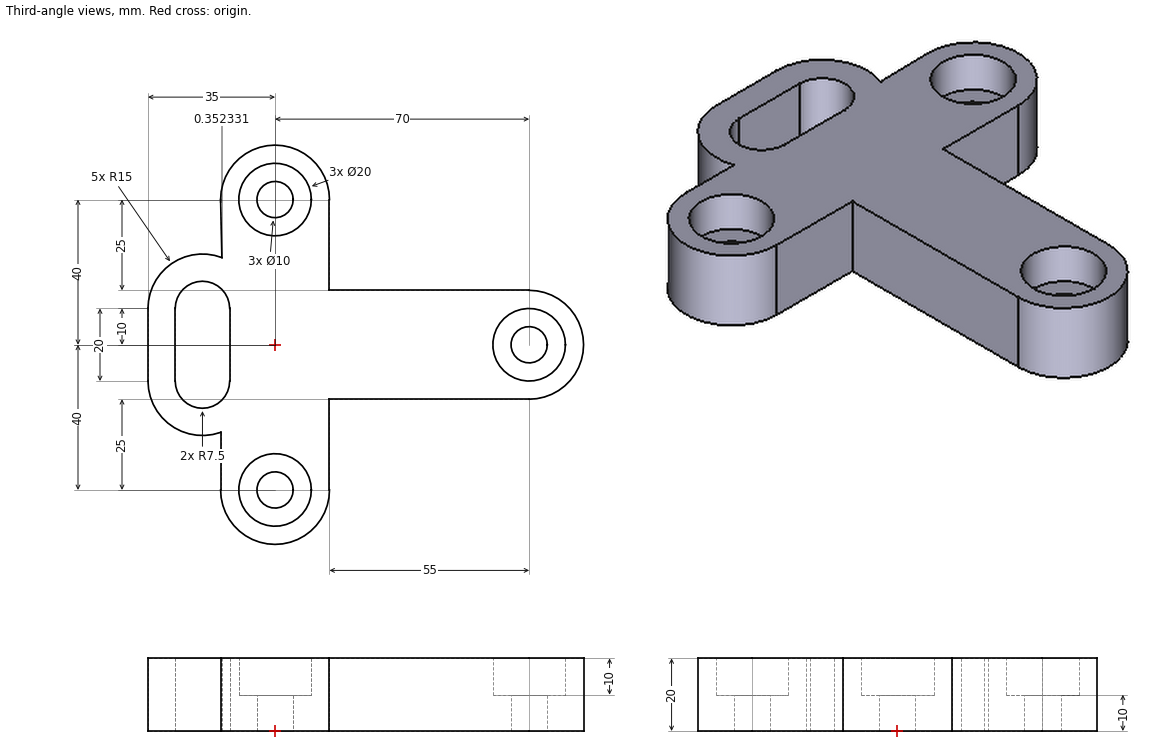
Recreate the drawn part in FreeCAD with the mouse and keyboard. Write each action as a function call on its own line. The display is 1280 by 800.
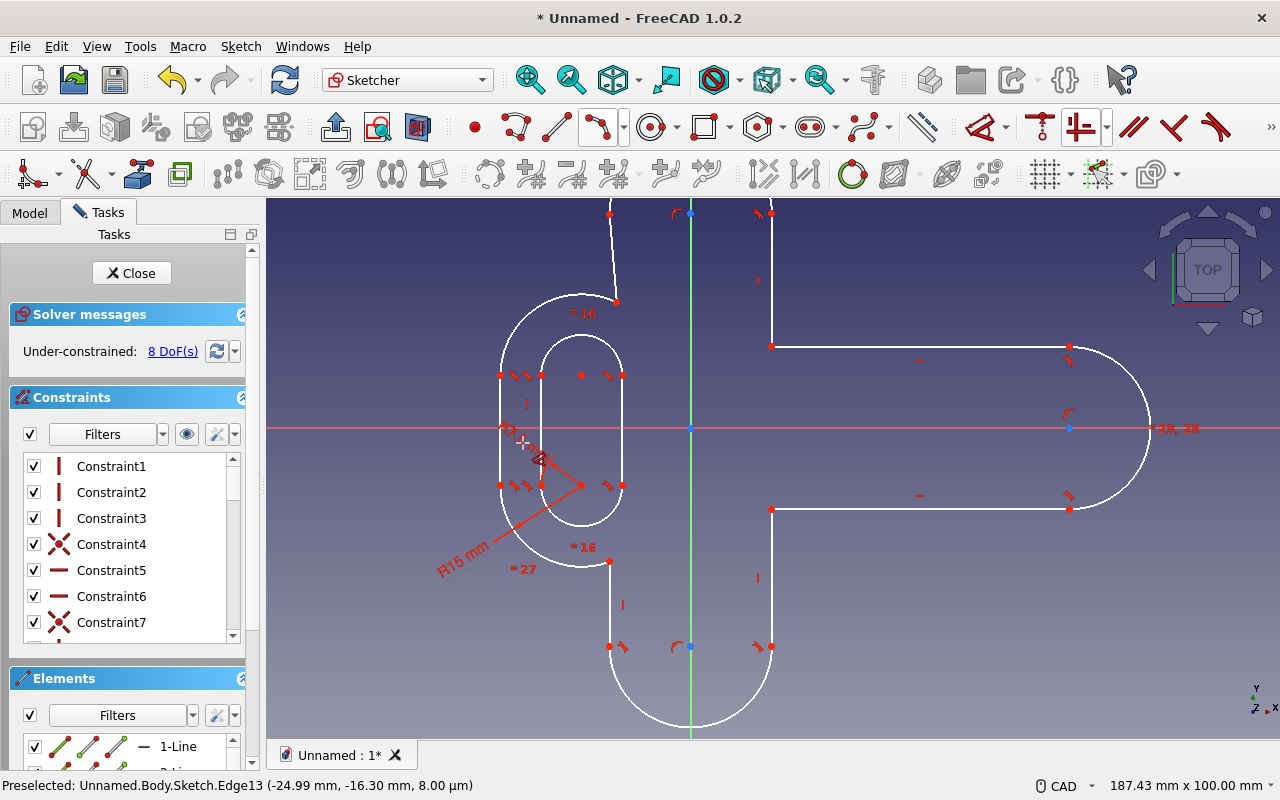
click(500, 409)
click(466, 405)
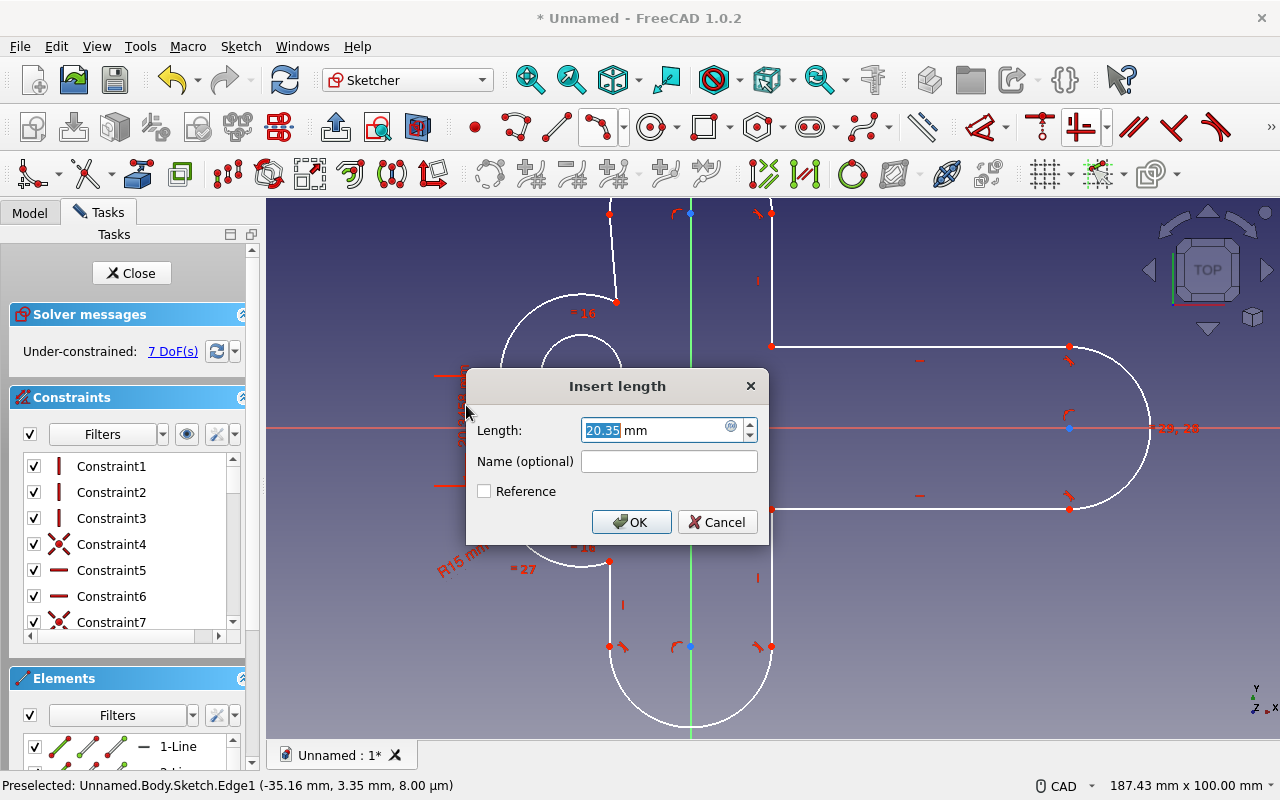
text(20)
key(Return)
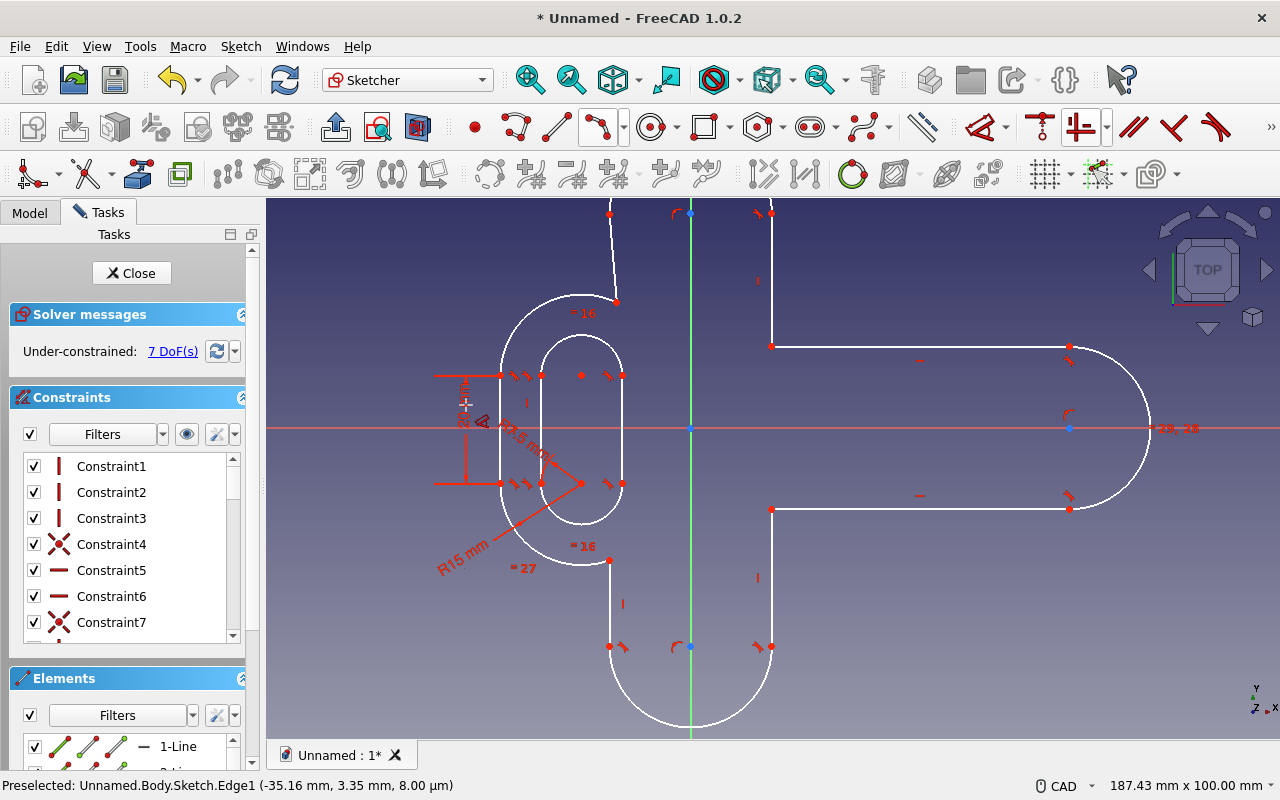
click(772, 605)
click(738, 578)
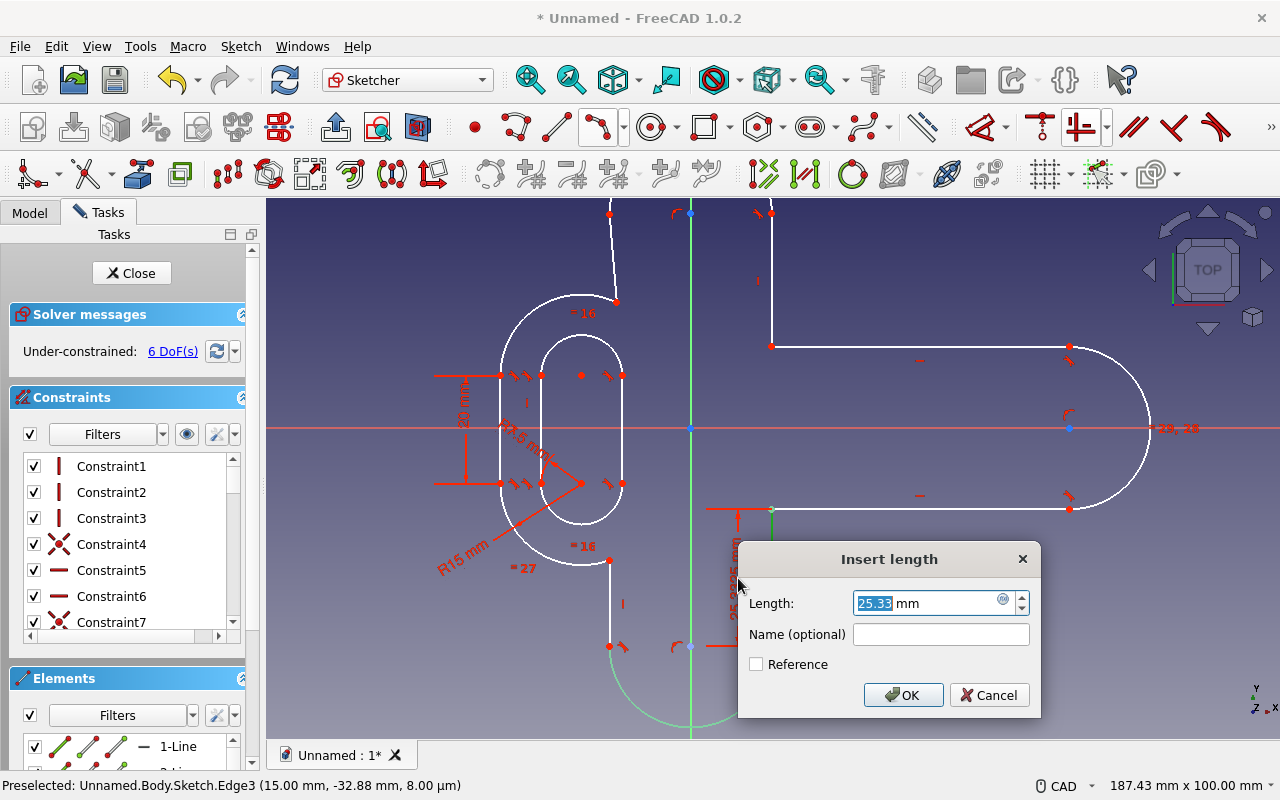
text(25)
key(Return)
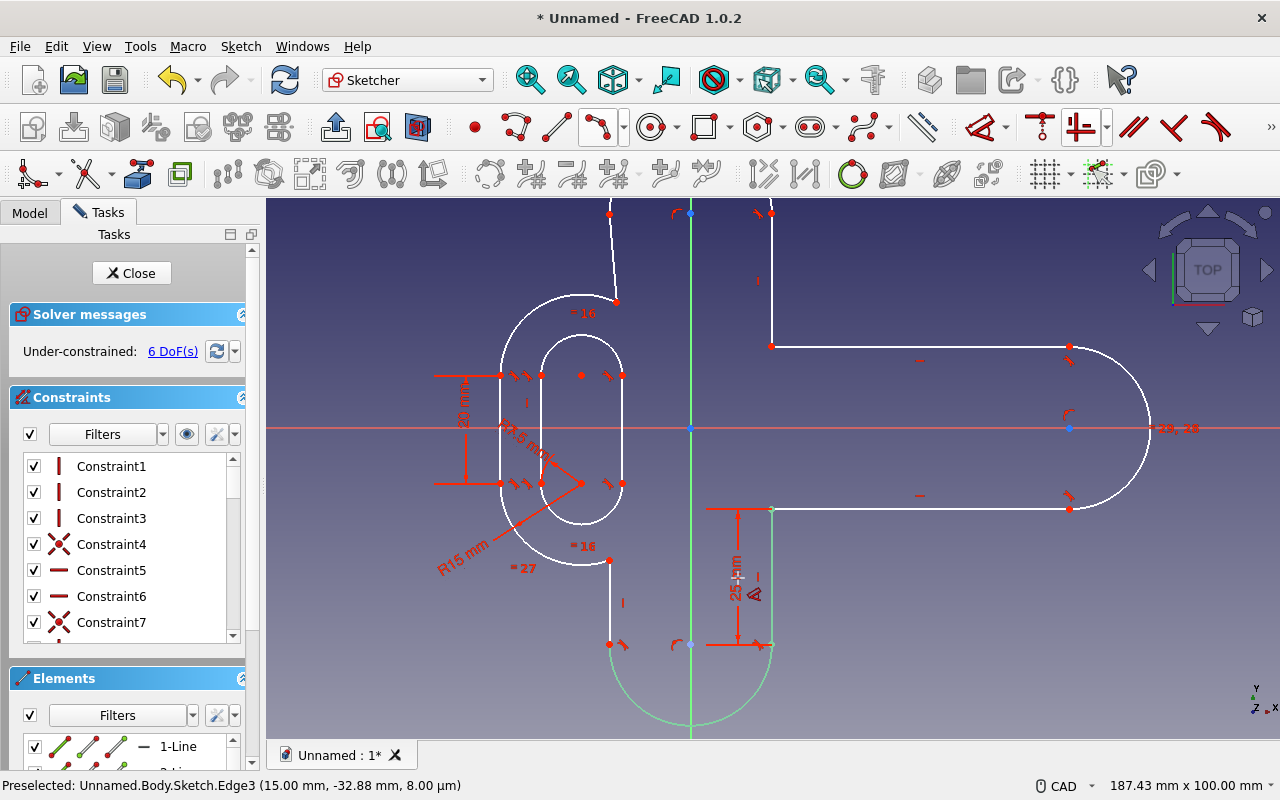
click(861, 509)
click(921, 543)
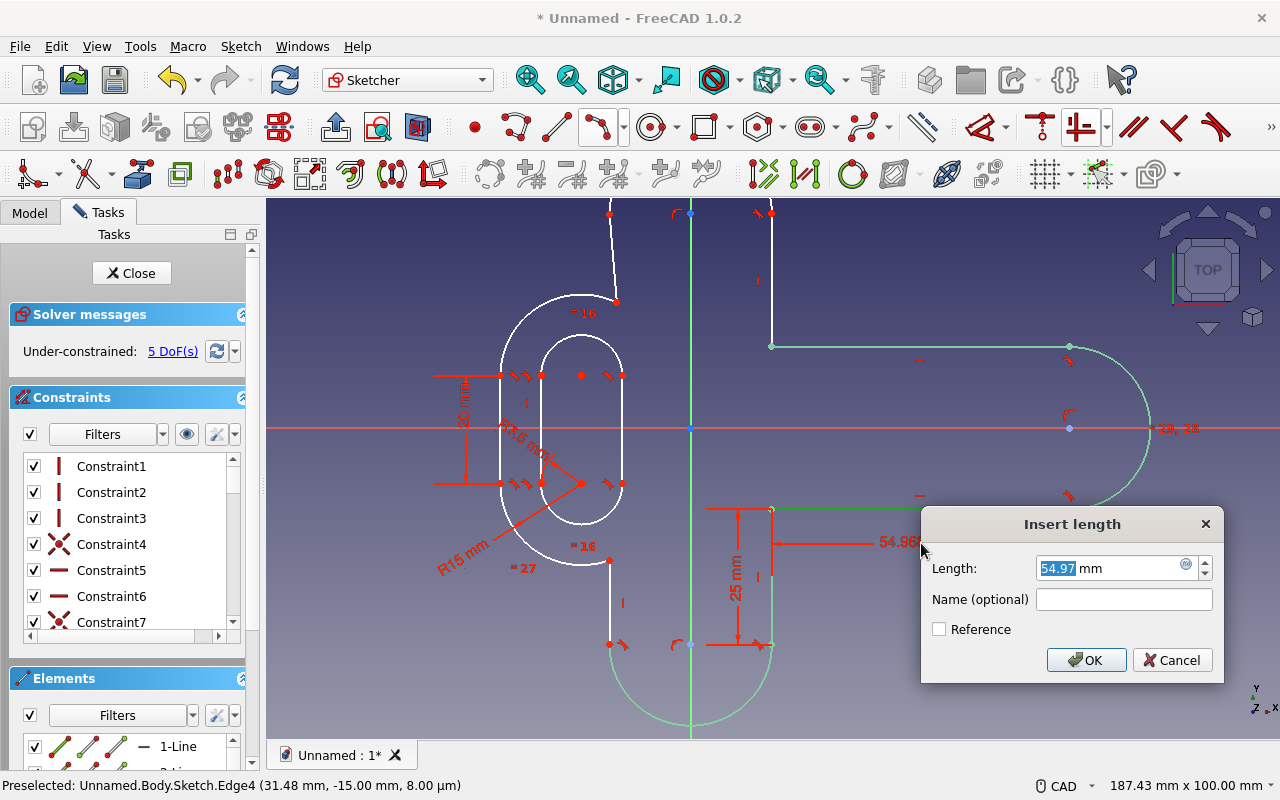
text(55)
key(Return)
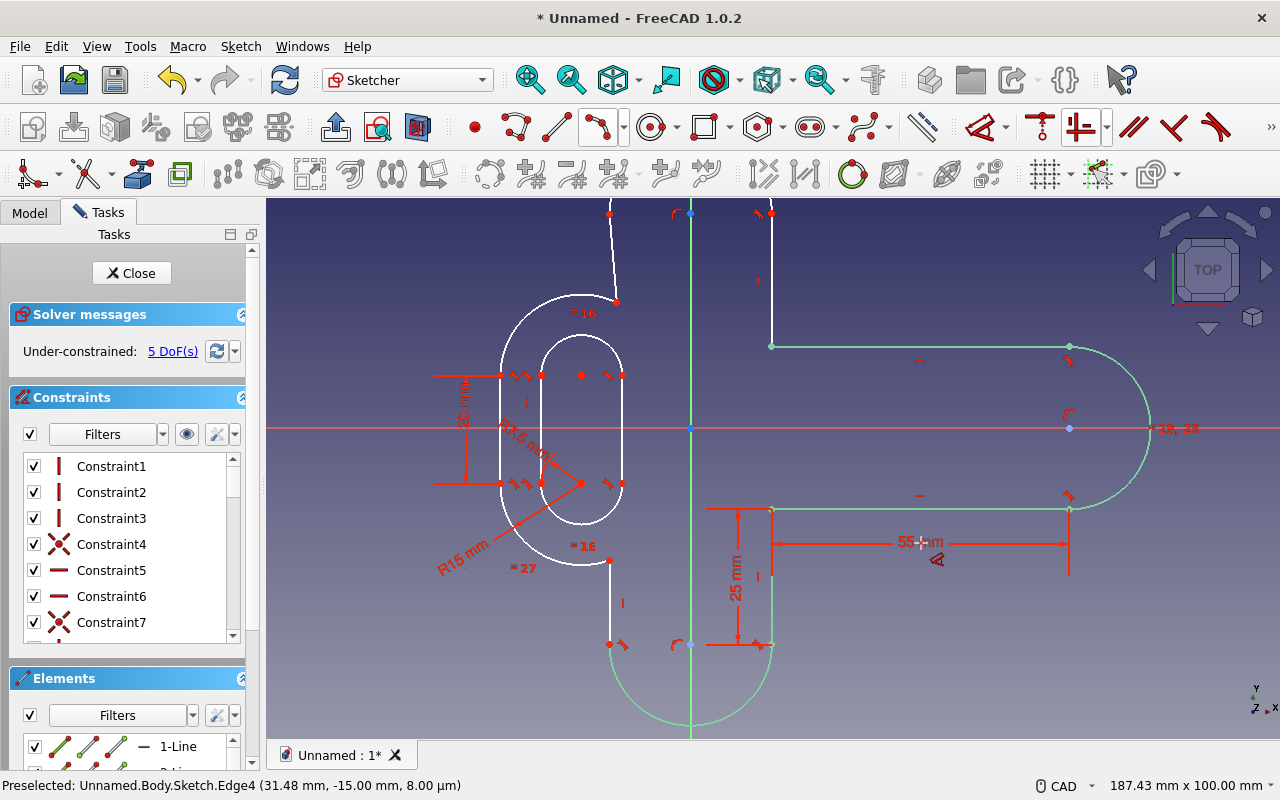
click(772, 307)
click(738, 286)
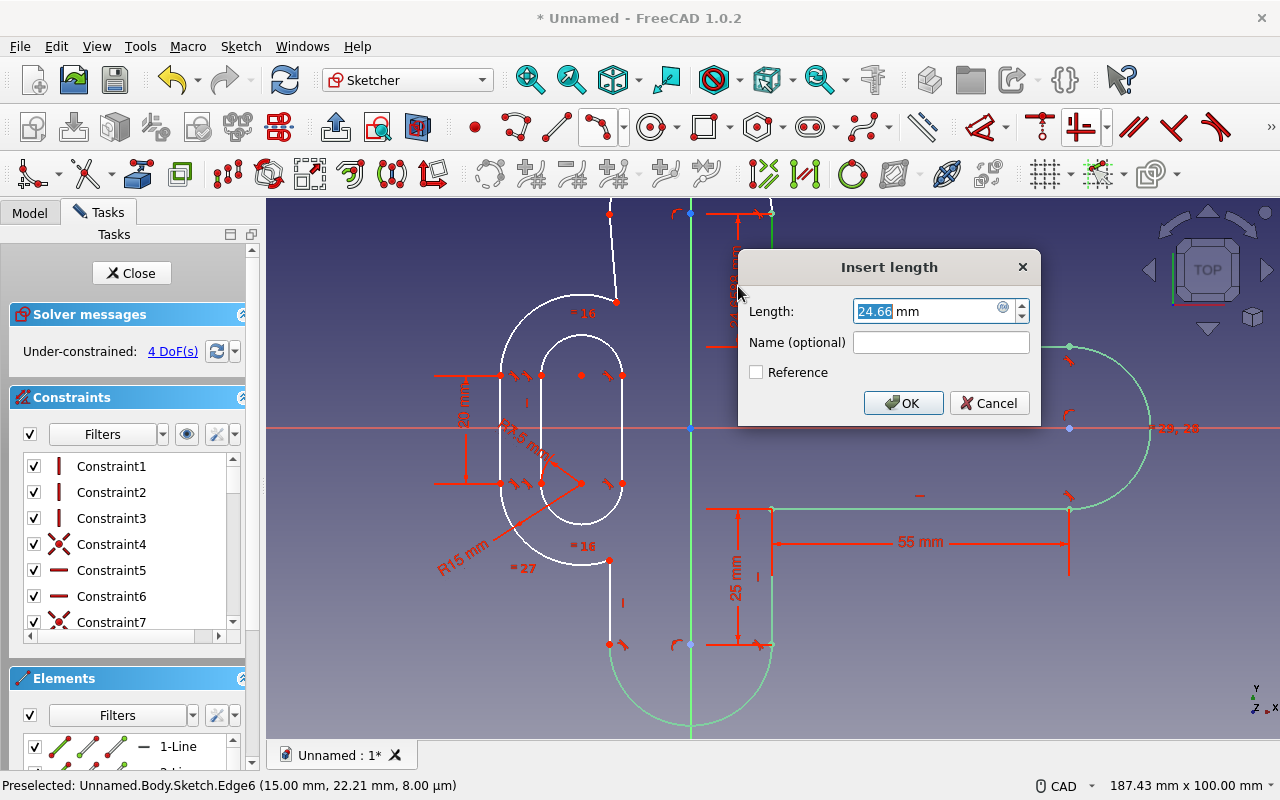
text(25)
key(Return)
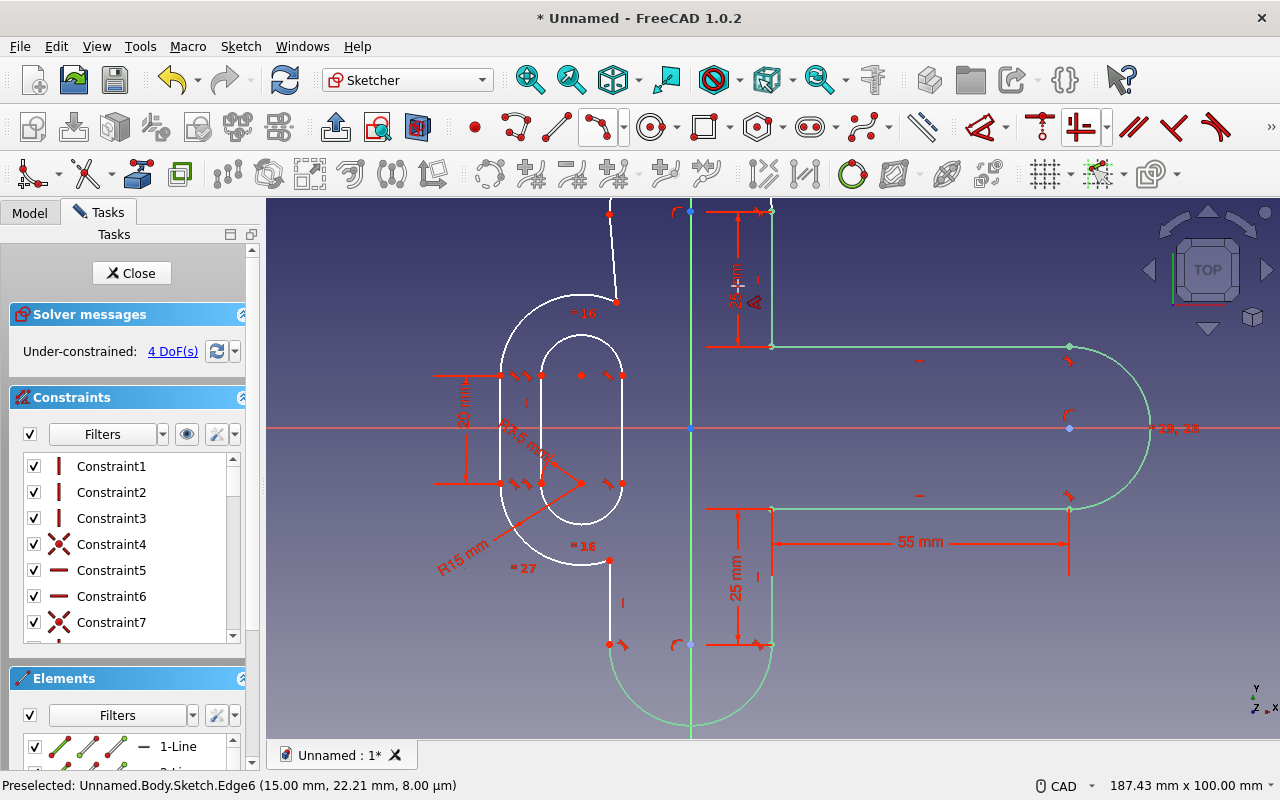
click(500, 376)
click(639, 342)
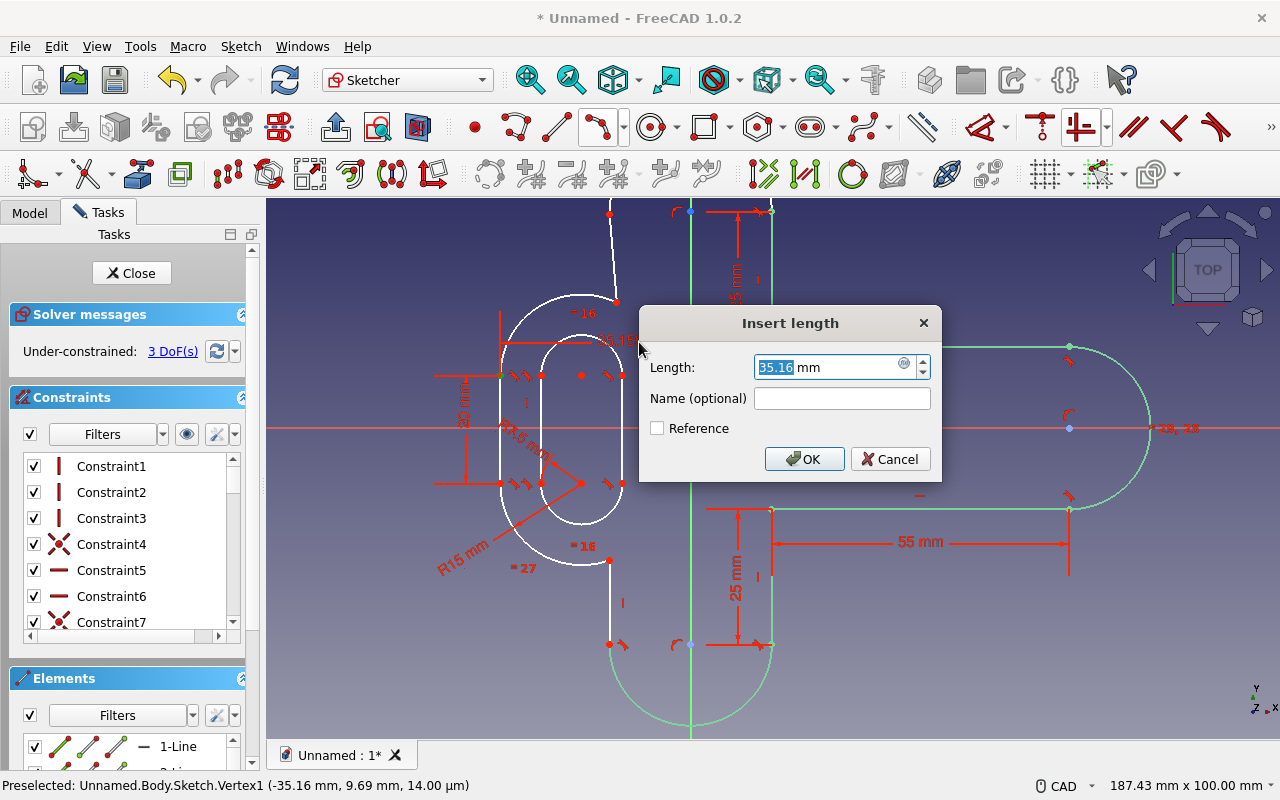
text(35)
key(Return)